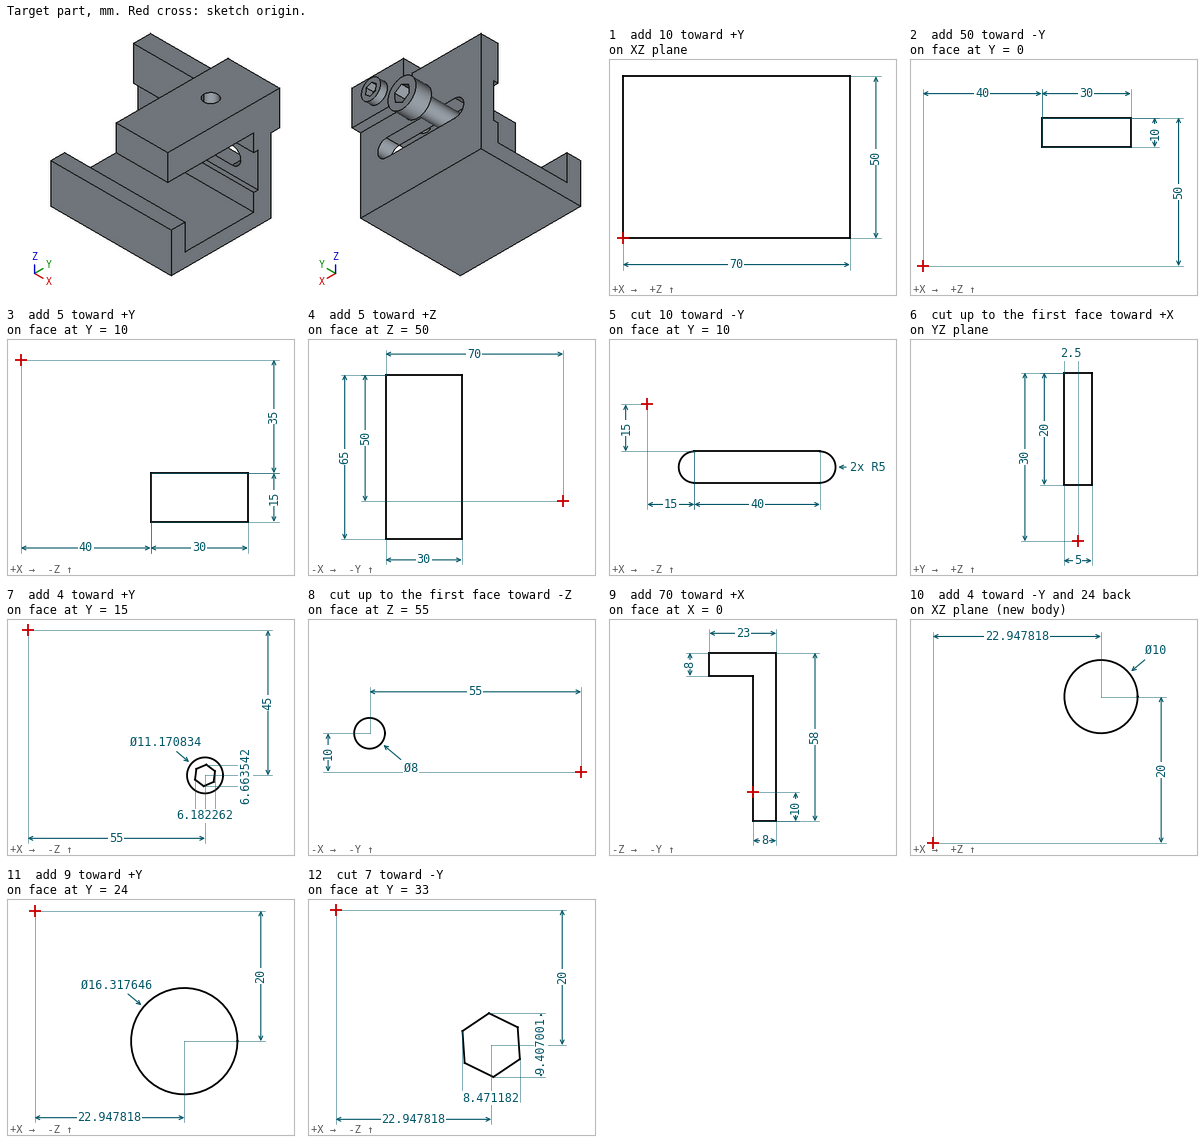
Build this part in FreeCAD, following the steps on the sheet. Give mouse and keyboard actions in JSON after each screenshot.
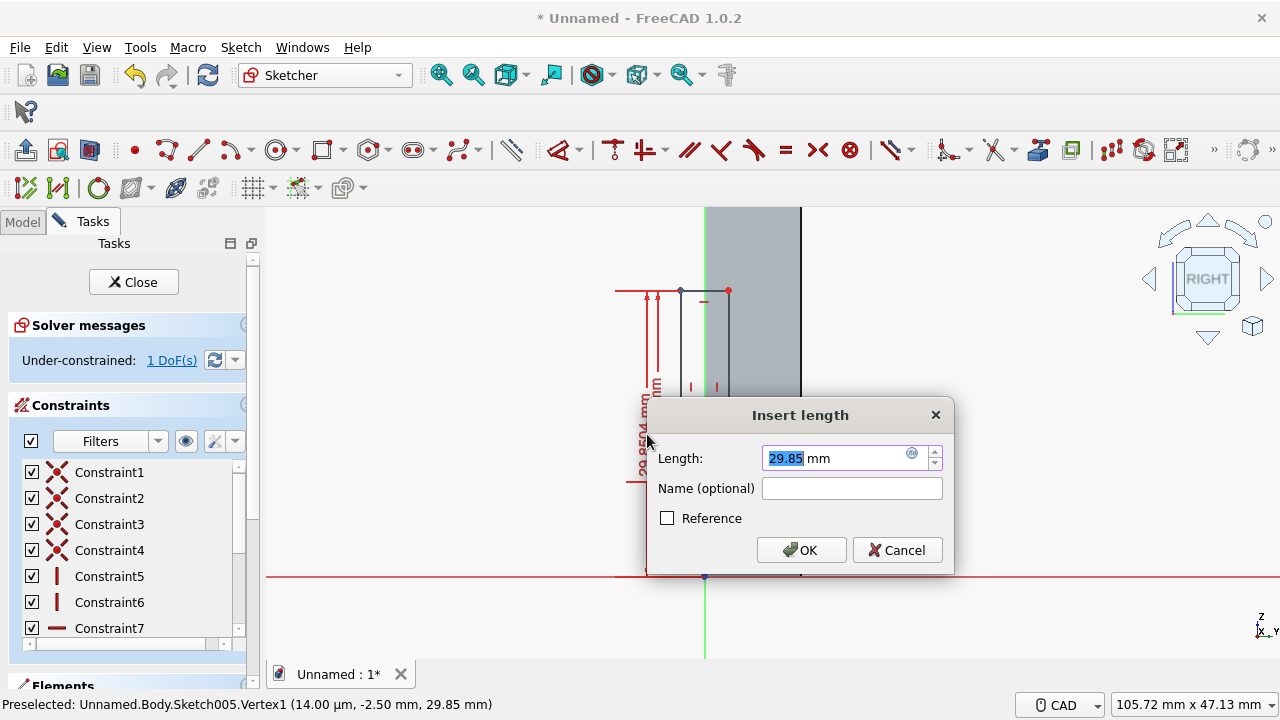
{"action": "type", "text": "30"}
{"action": "key", "text": "Return"}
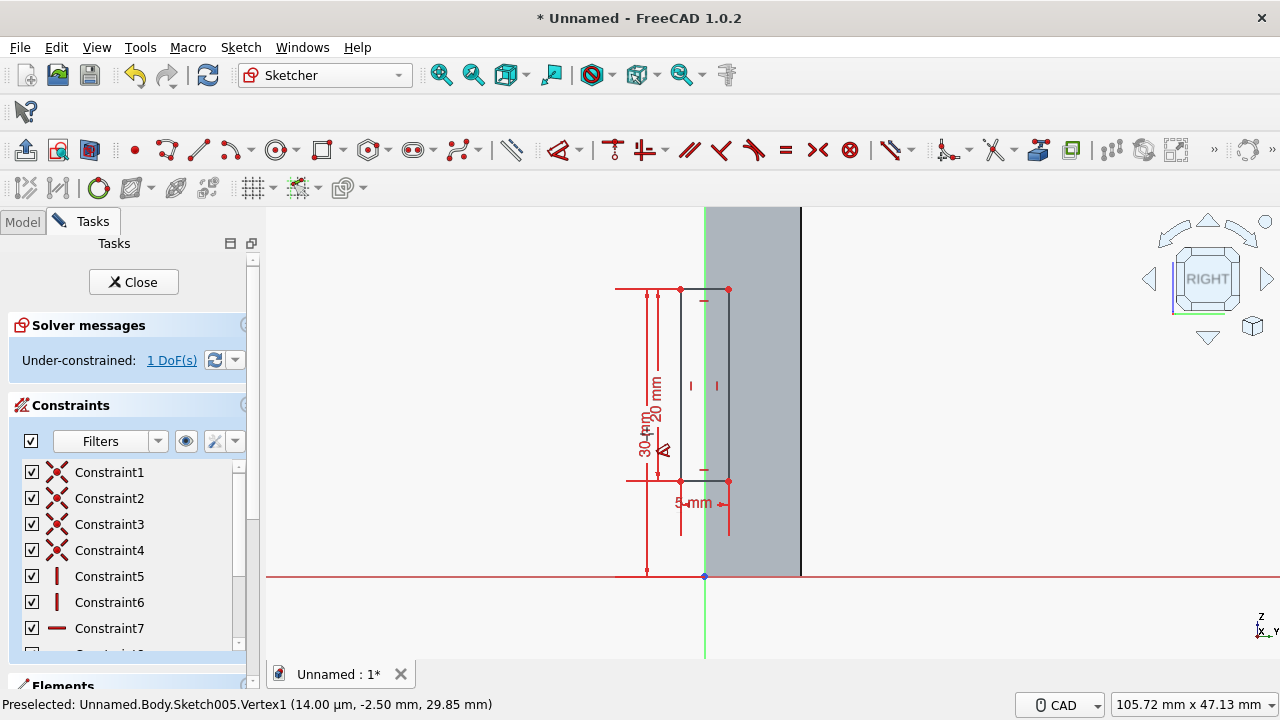
{"action": "scroll", "coordinate": [681, 289], "scroll_direction": "up", "scroll_amount": 3}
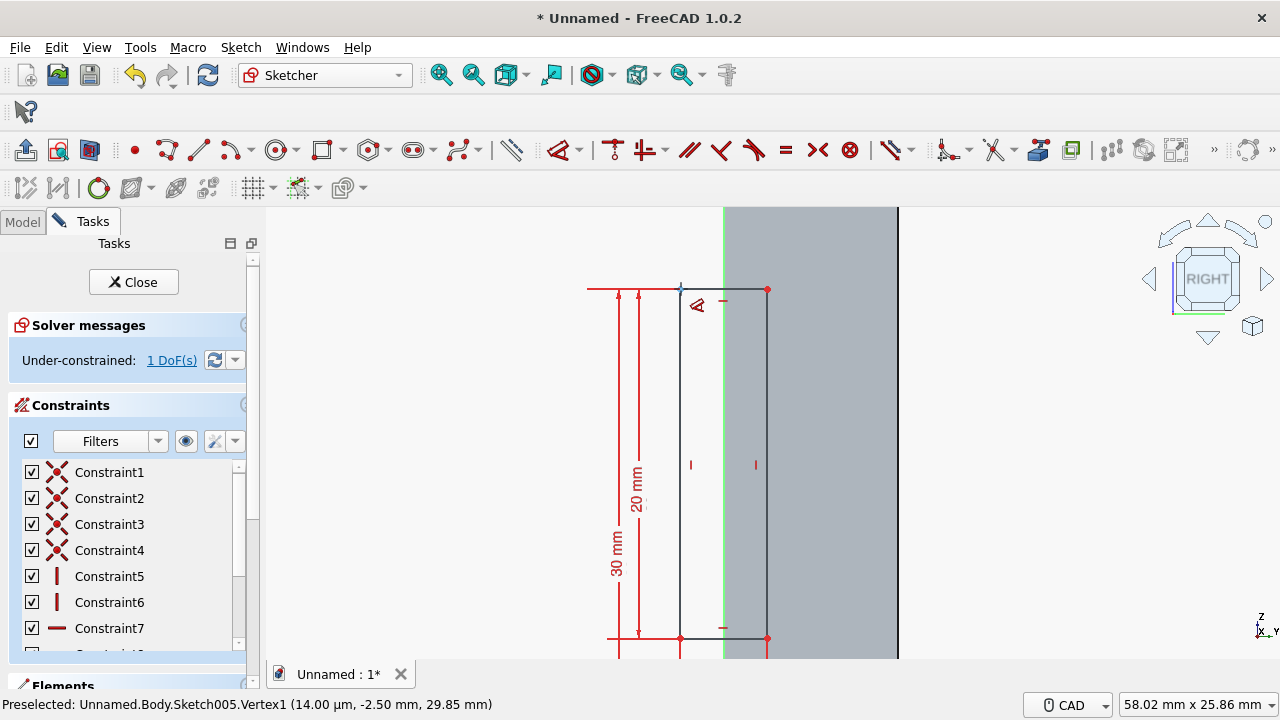
{"action": "left_click", "coordinate": [680, 289]}
{"action": "left_click", "coordinate": [702, 255]}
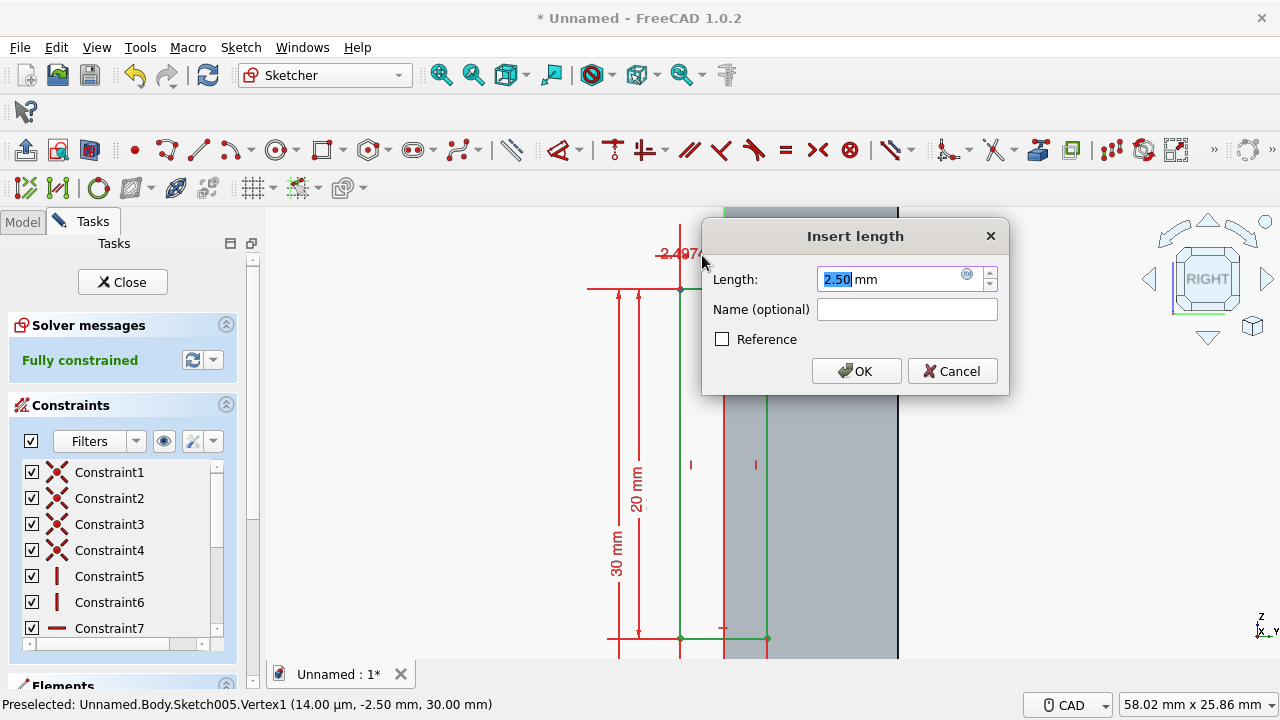
{"action": "type", "text": "2.5"}
{"action": "key", "text": "Return"}
{"action": "key", "text": "Escape"}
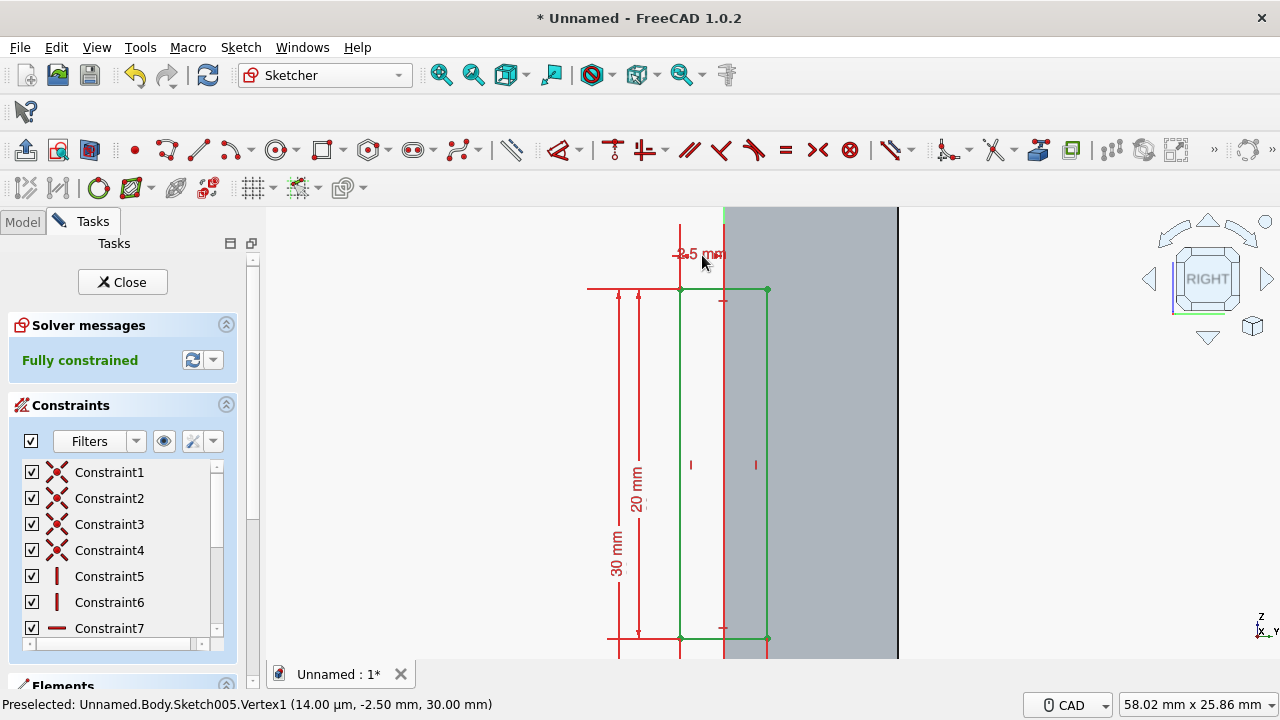
{"action": "left_click", "coordinate": [123, 282]}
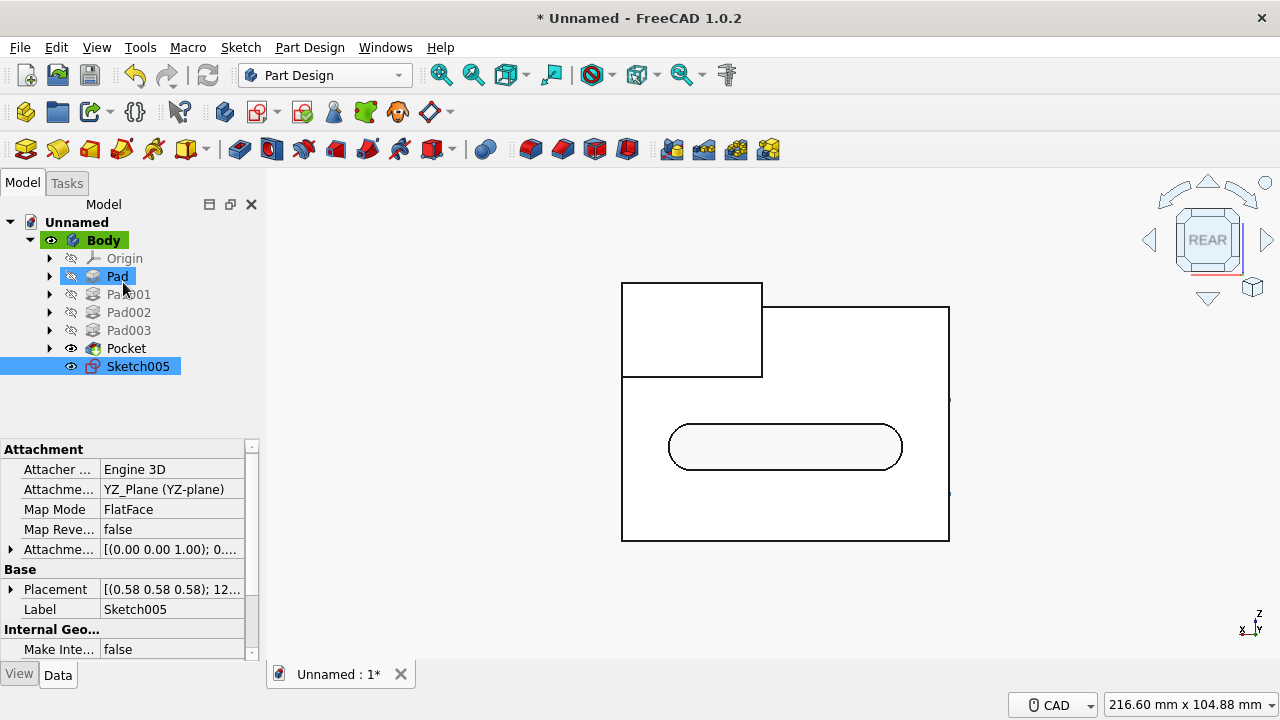
{"action": "left_click", "coordinate": [240, 150]}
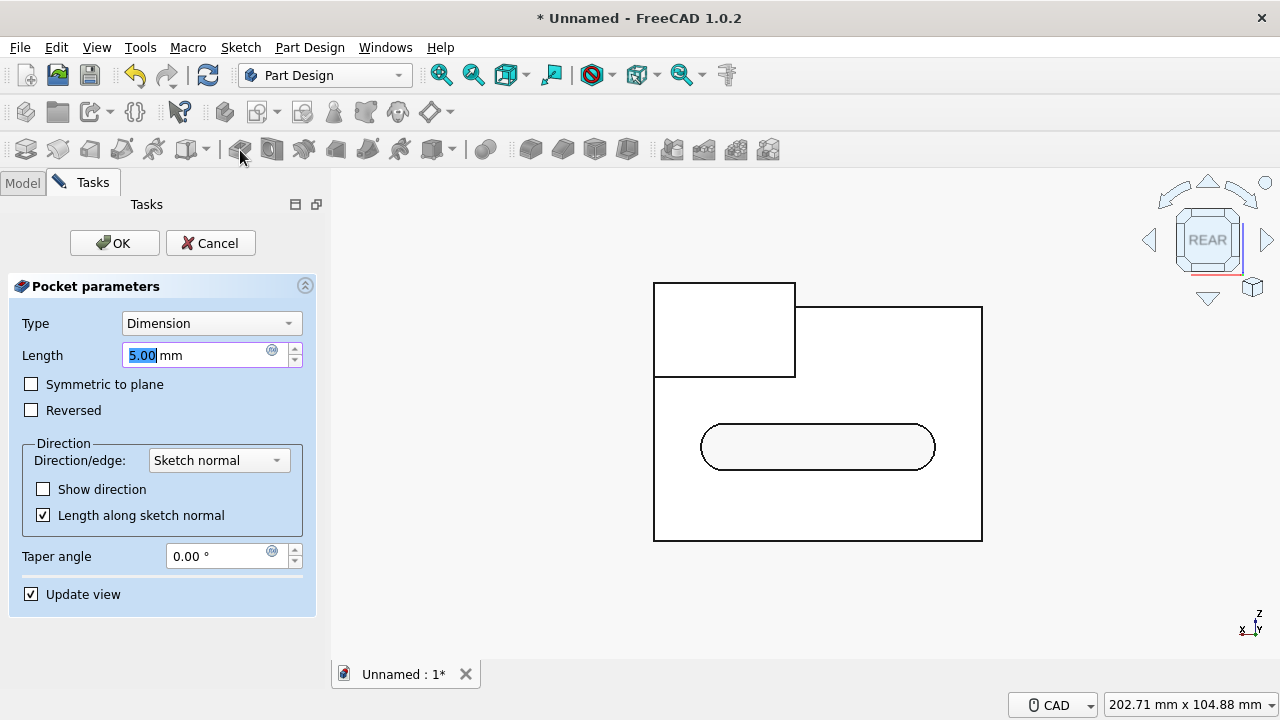
{"action": "left_click", "coordinate": [212, 324]}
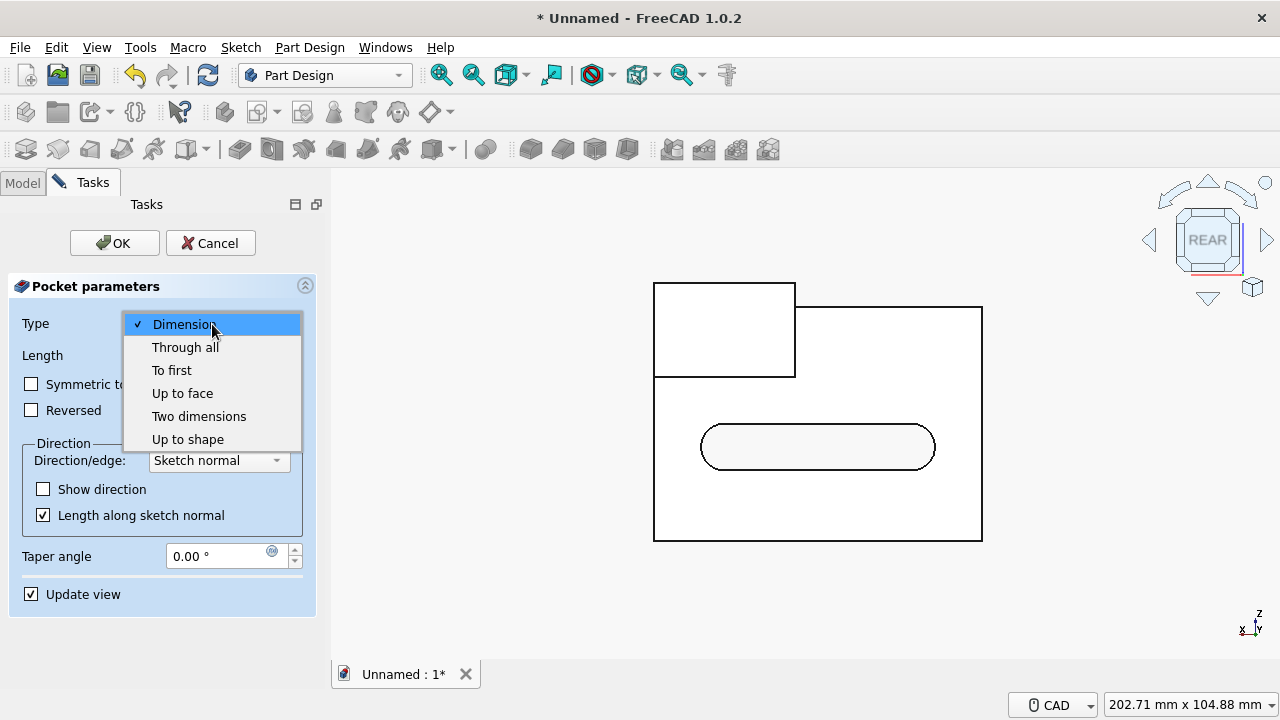
{"action": "left_click", "coordinate": [212, 370]}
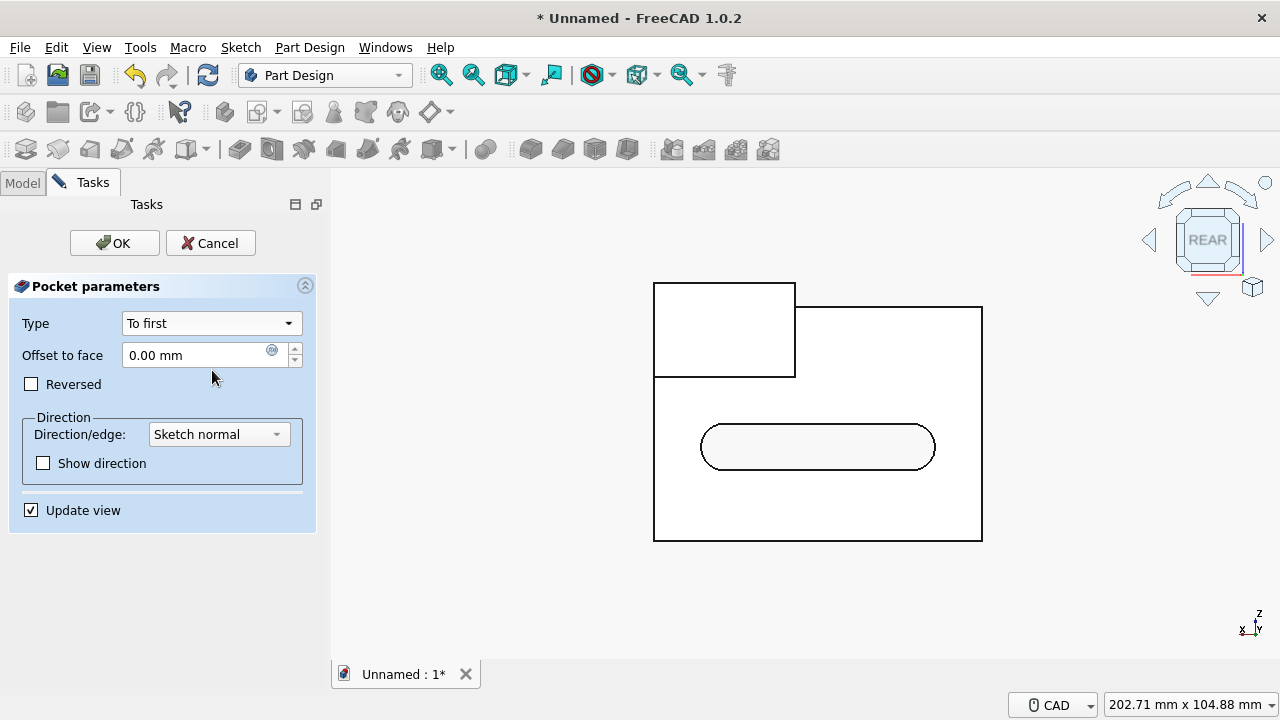
{"action": "left_click", "coordinate": [30, 384]}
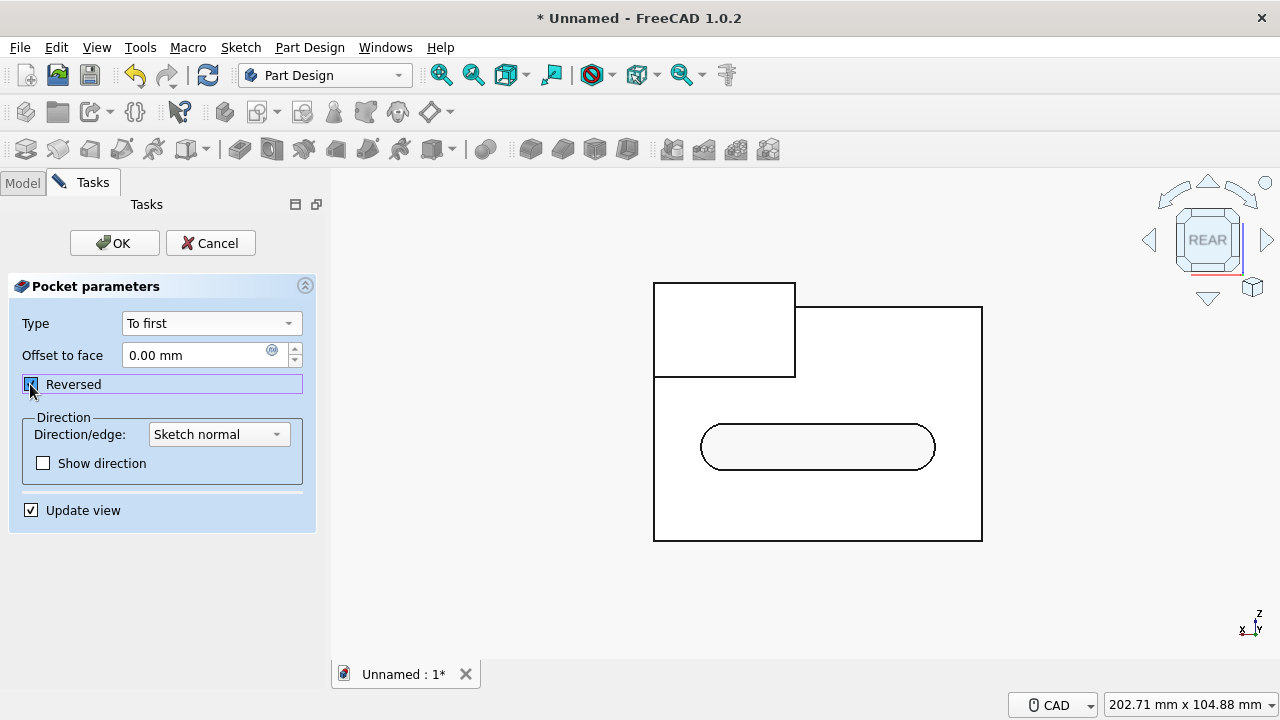
{"action": "left_click", "coordinate": [115, 243]}